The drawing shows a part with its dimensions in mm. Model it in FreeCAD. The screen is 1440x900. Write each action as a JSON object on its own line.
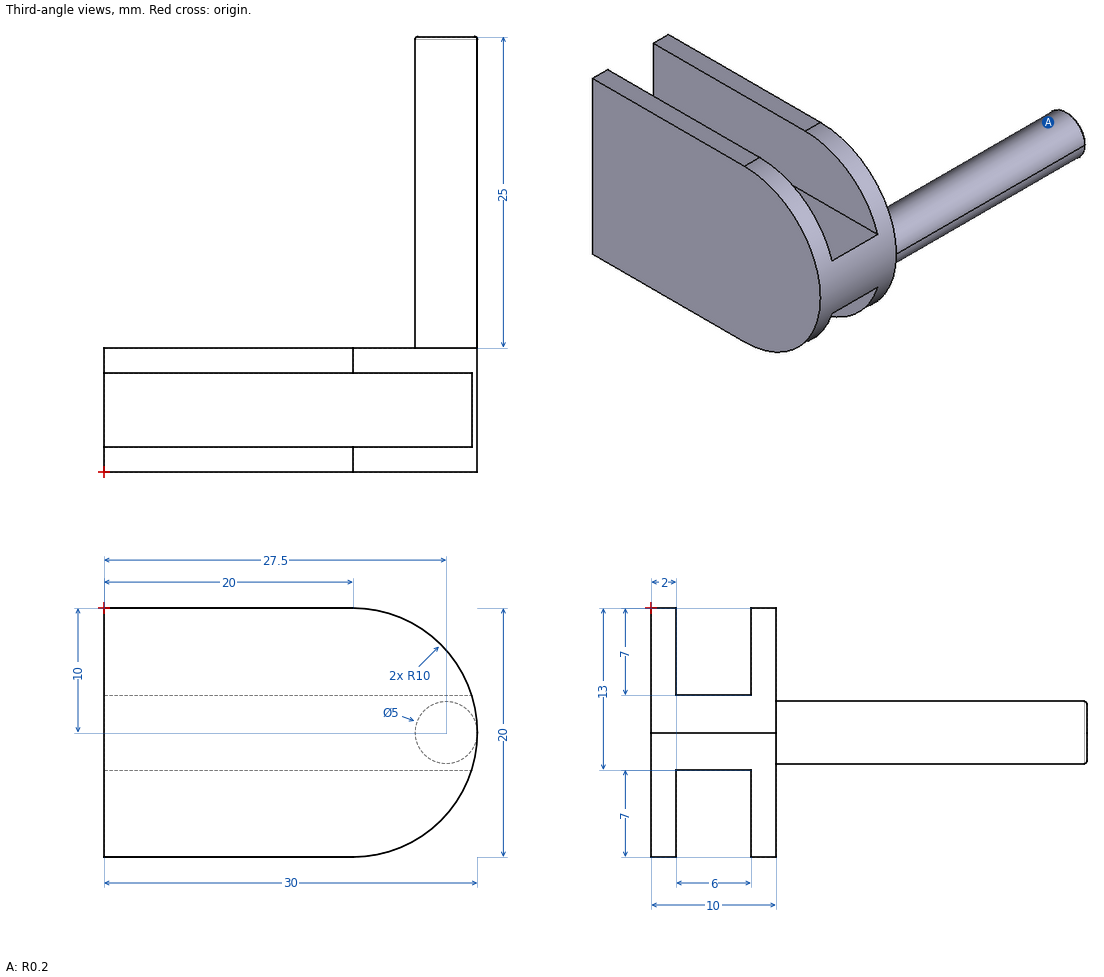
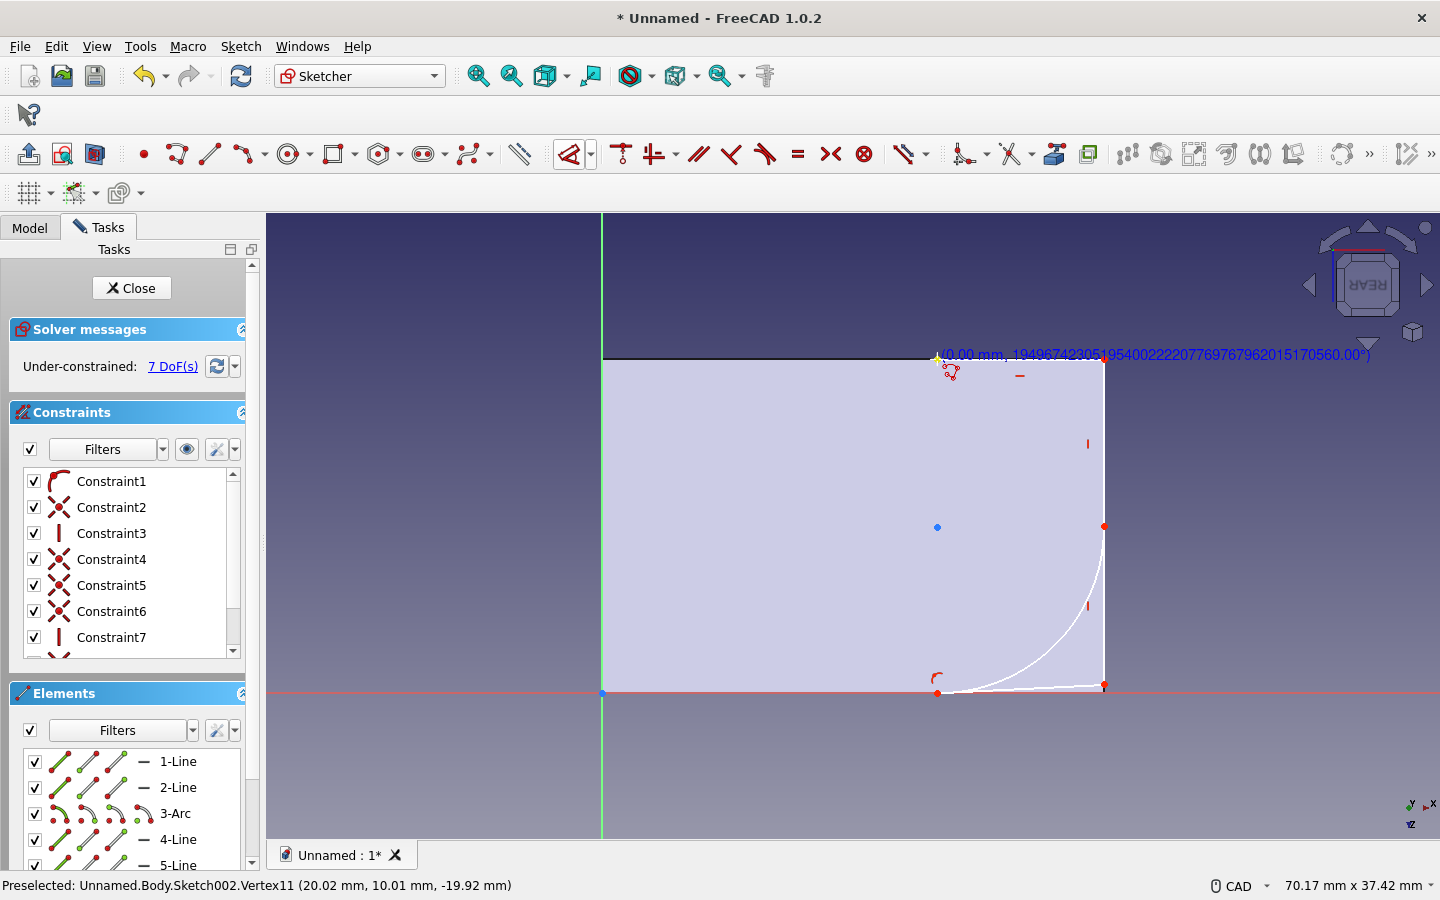
{"action": "left_click", "coordinate": [242, 154]}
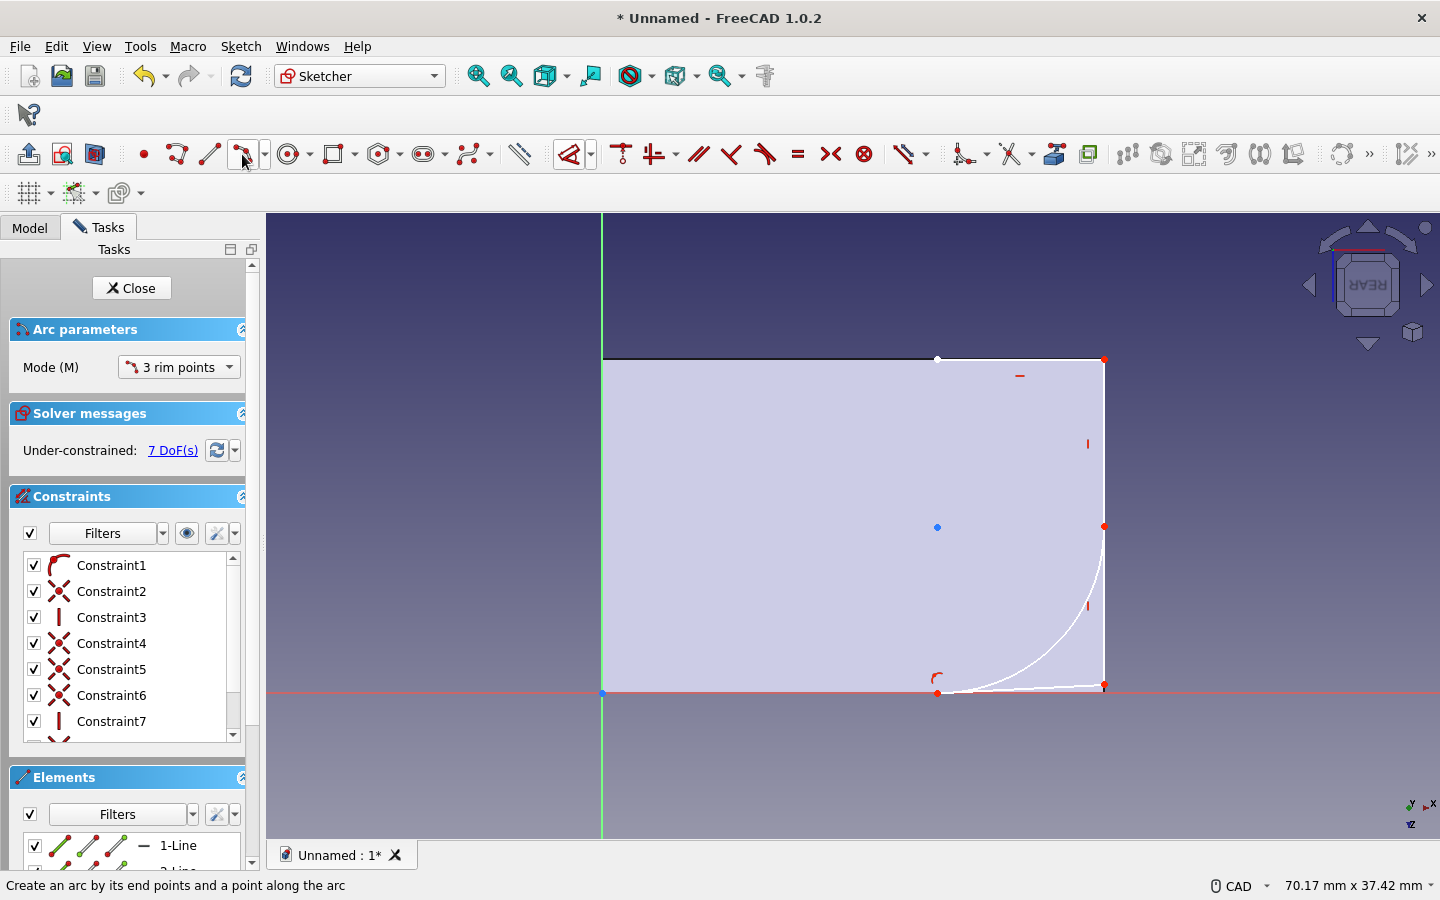
{"action": "left_click", "coordinate": [937, 360]}
{"action": "left_click", "coordinate": [1104, 527]}
{"action": "left_click", "coordinate": [1055, 408]}
{"action": "key", "text": "Escape"}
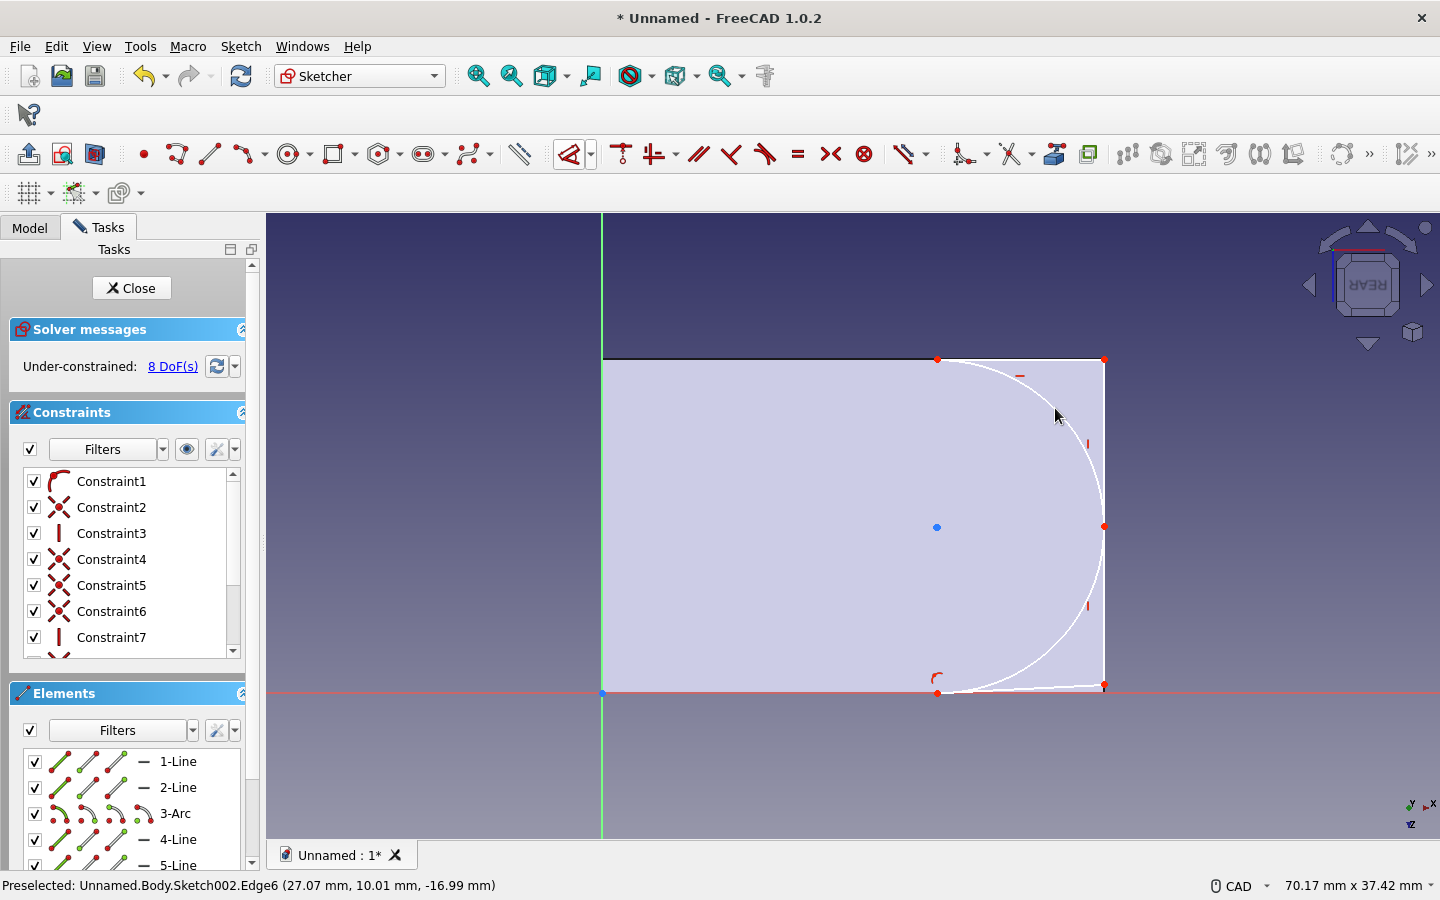
{"action": "scroll", "coordinate": [1004, 690], "scroll_direction": "up", "scroll_amount": 2}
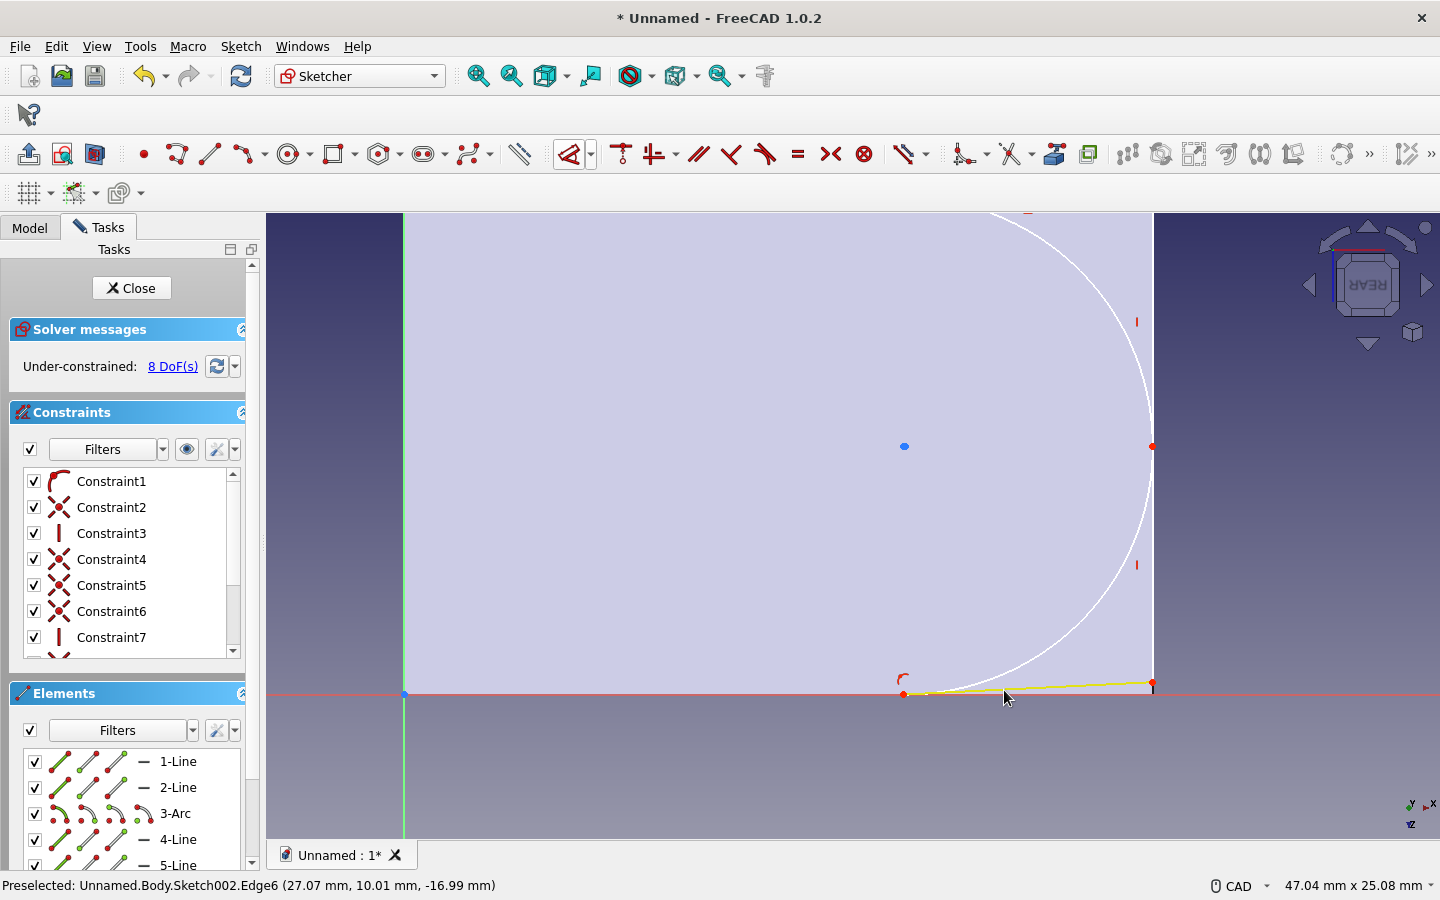
{"action": "left_click", "coordinate": [1003, 690]}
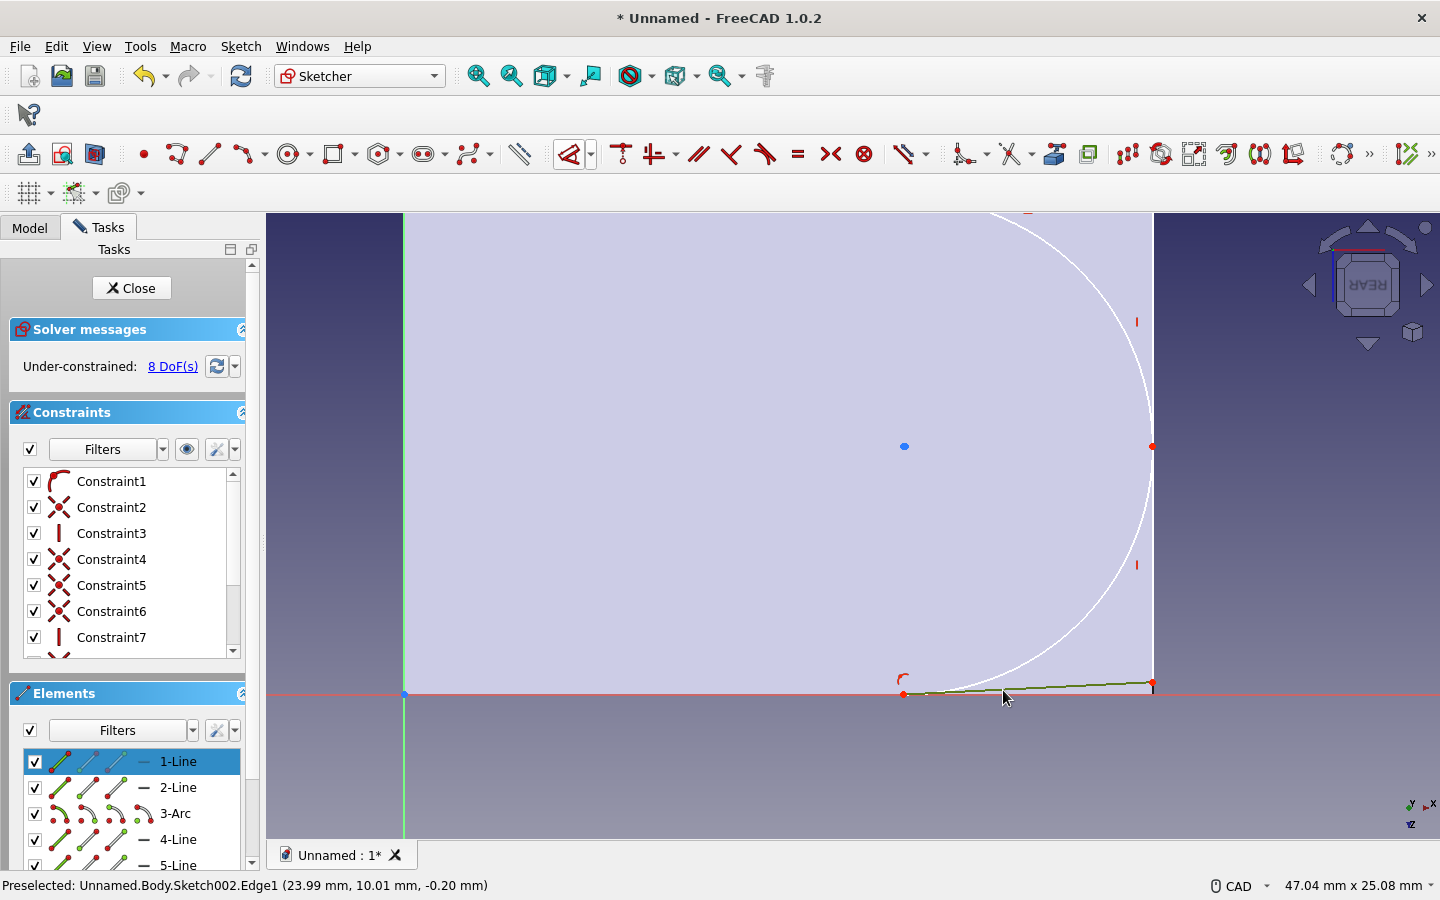
{"action": "left_click", "coordinate": [1017, 668]}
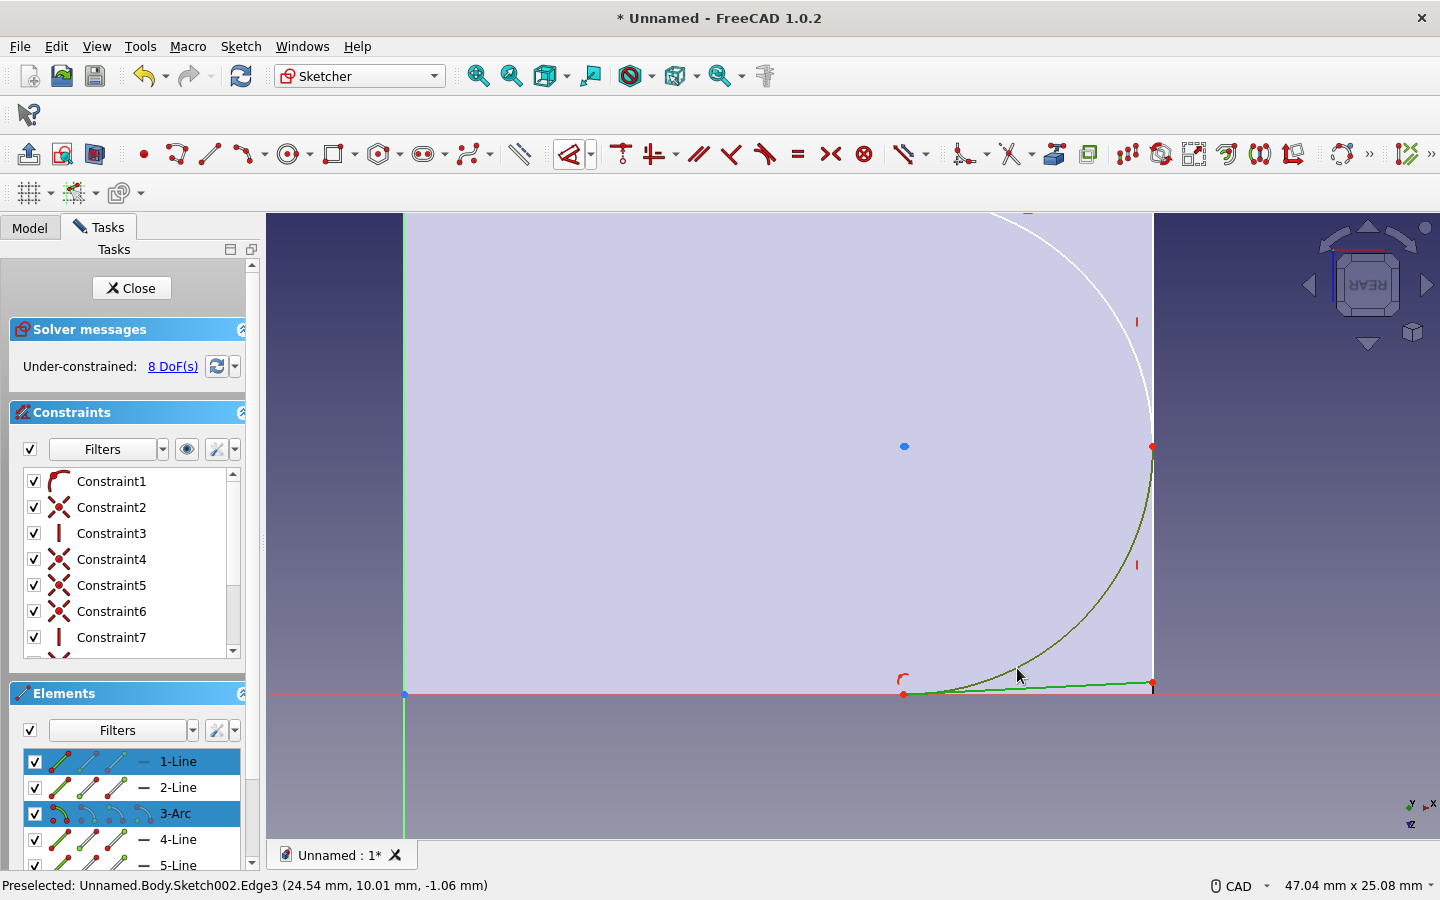
{"action": "left_click", "coordinate": [765, 154]}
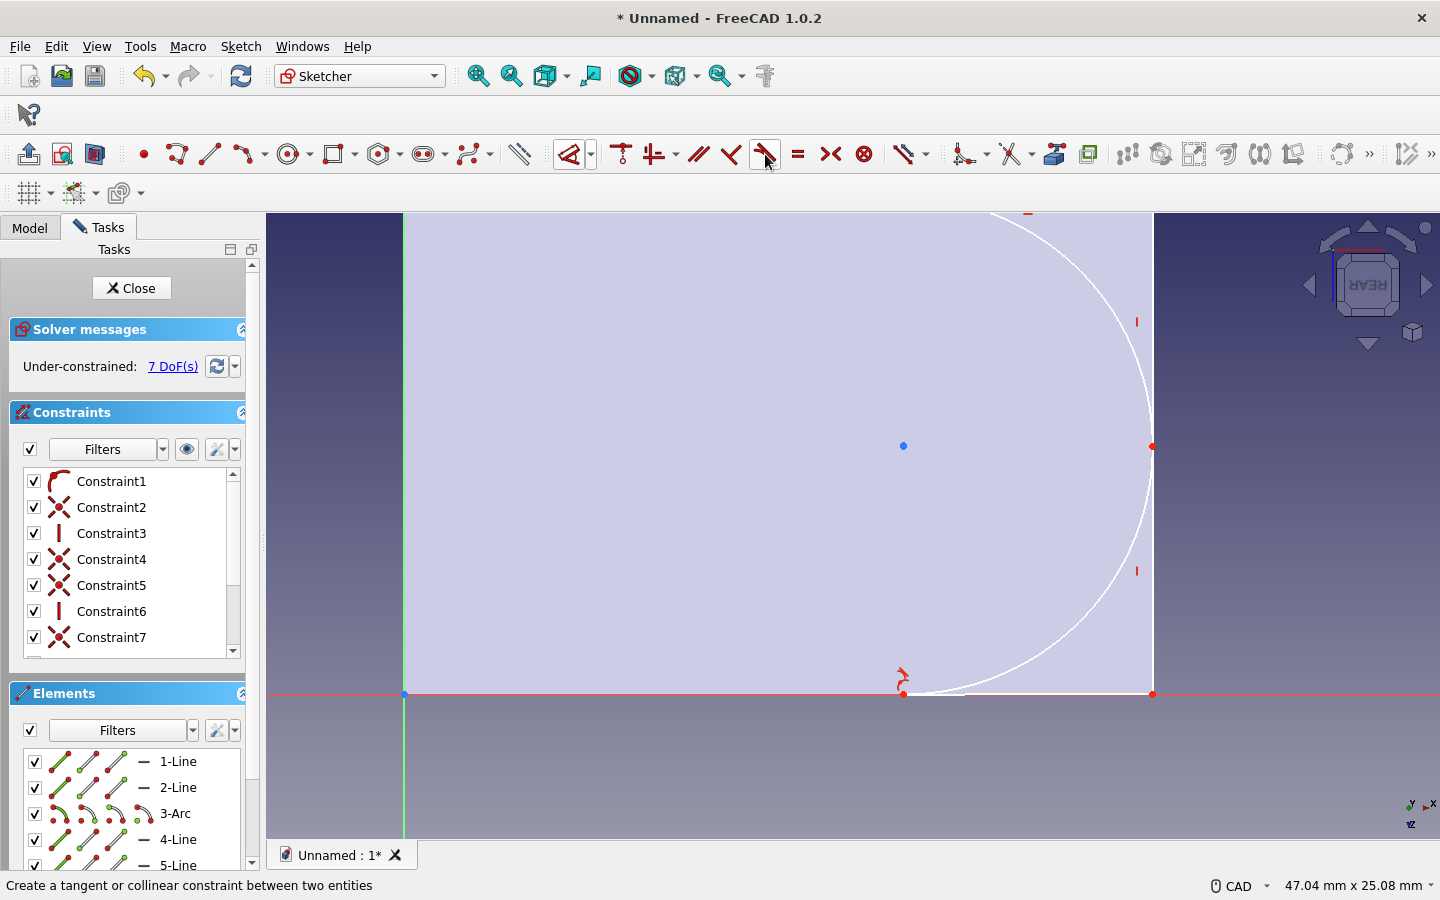
{"action": "left_click", "coordinate": [1153, 620]}